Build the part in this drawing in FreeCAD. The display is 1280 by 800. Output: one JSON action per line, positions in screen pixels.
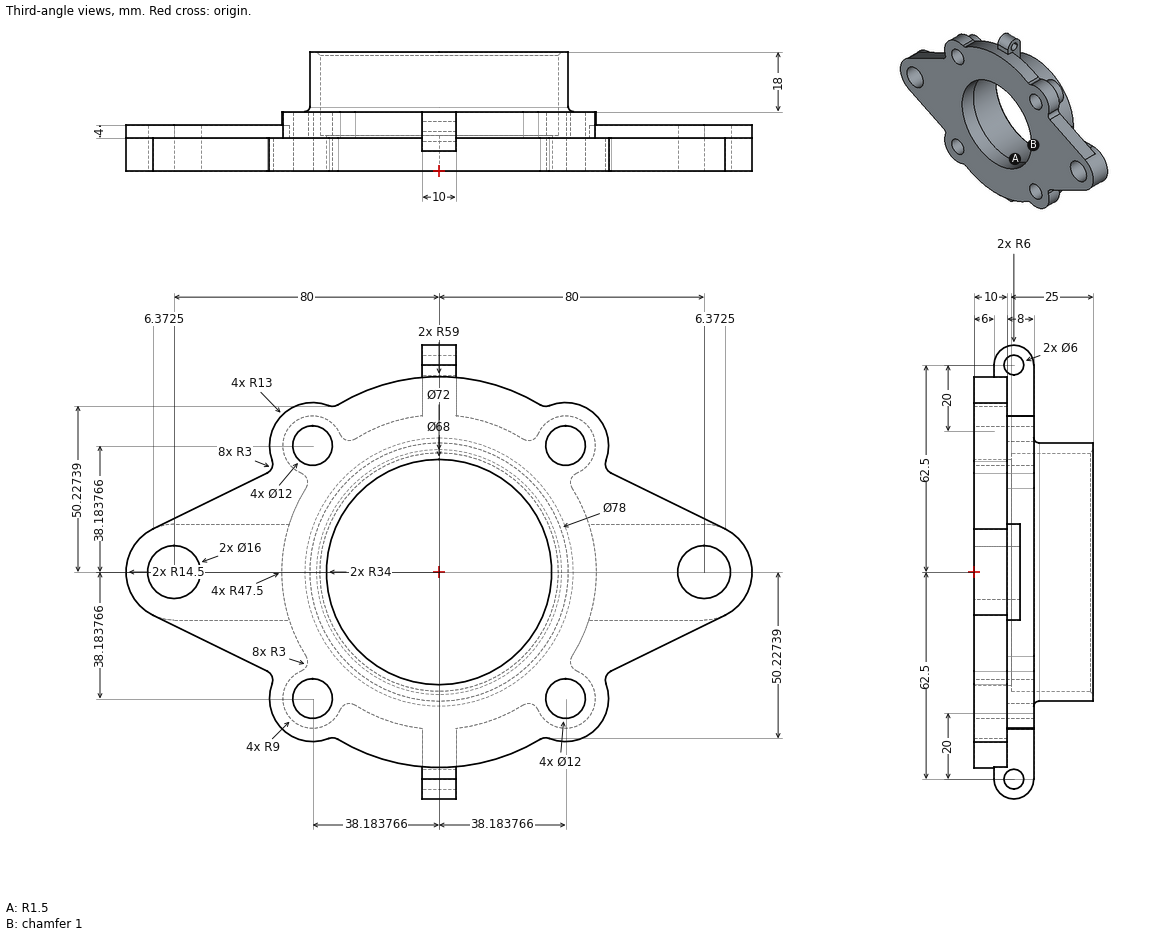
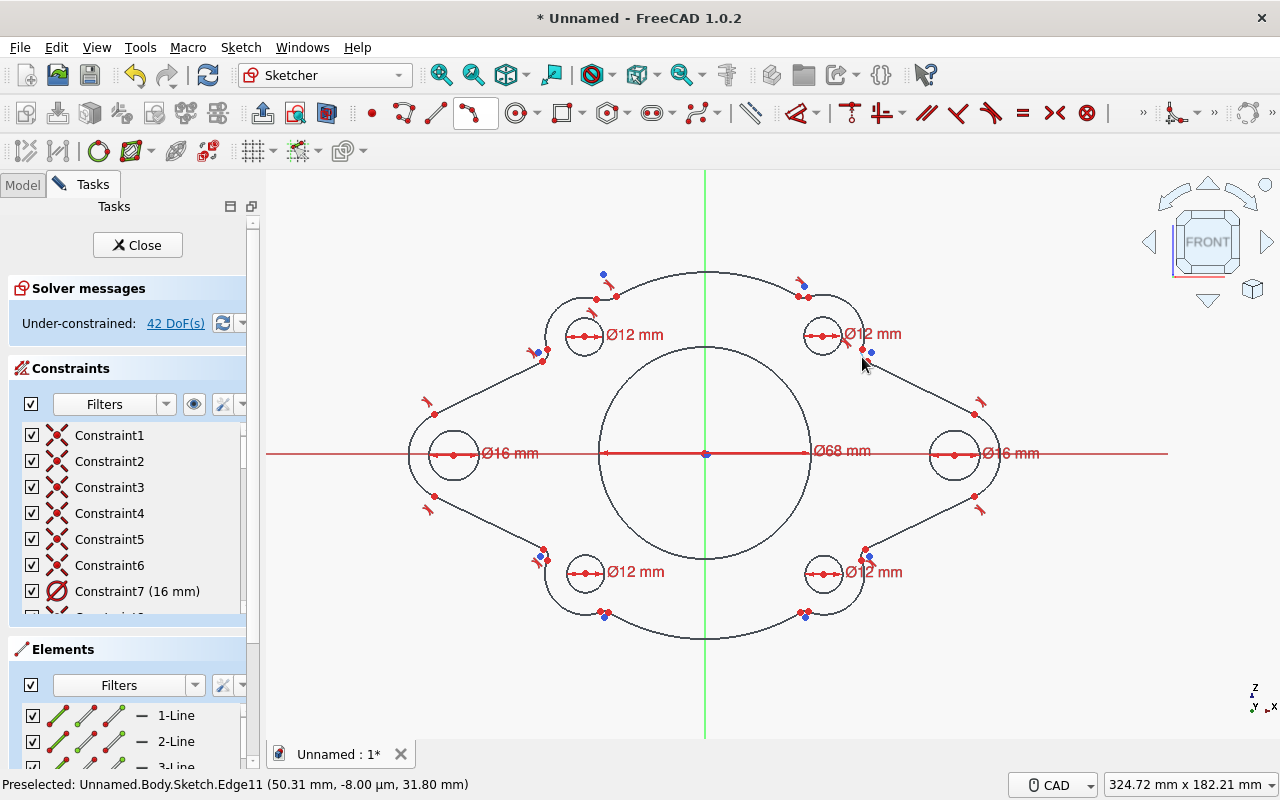
{"action": "scroll", "coordinate": [862, 554], "scroll_direction": "up", "scroll_amount": 4}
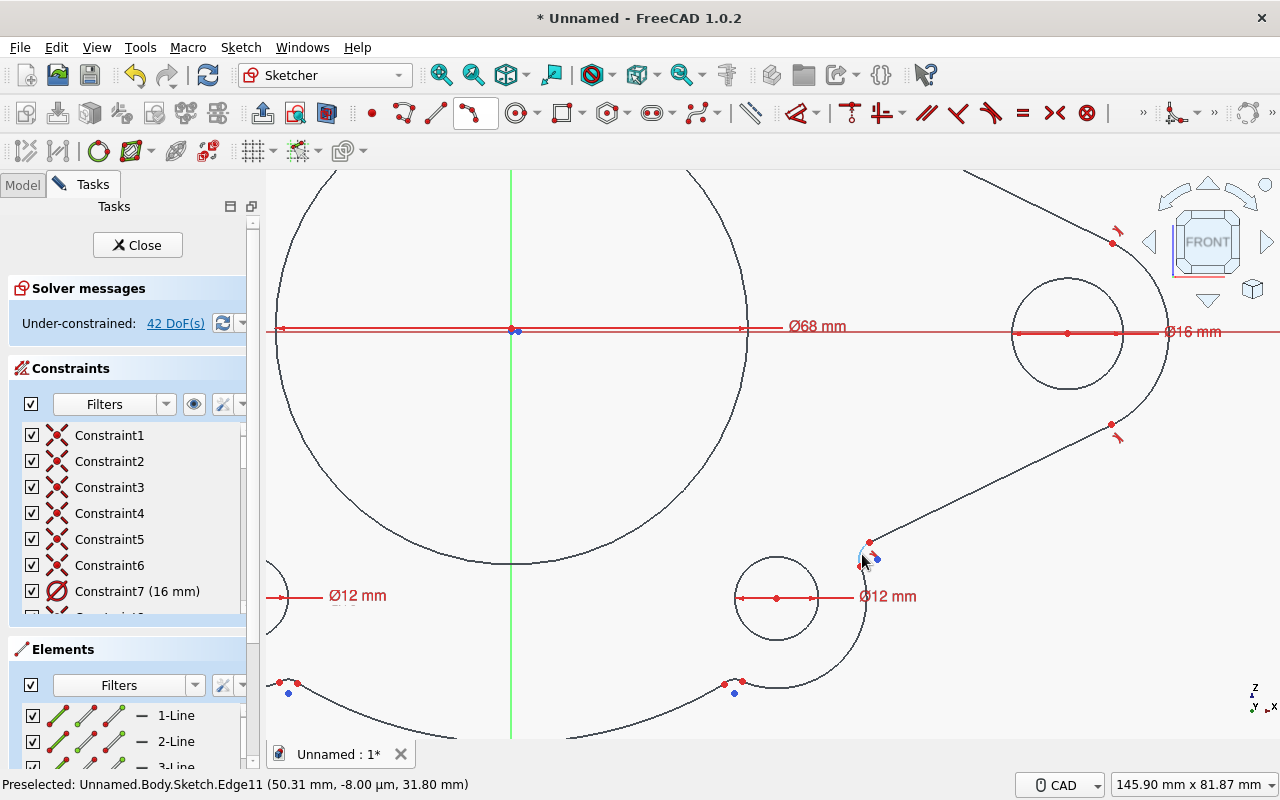
{"action": "left_click", "coordinate": [860, 553]}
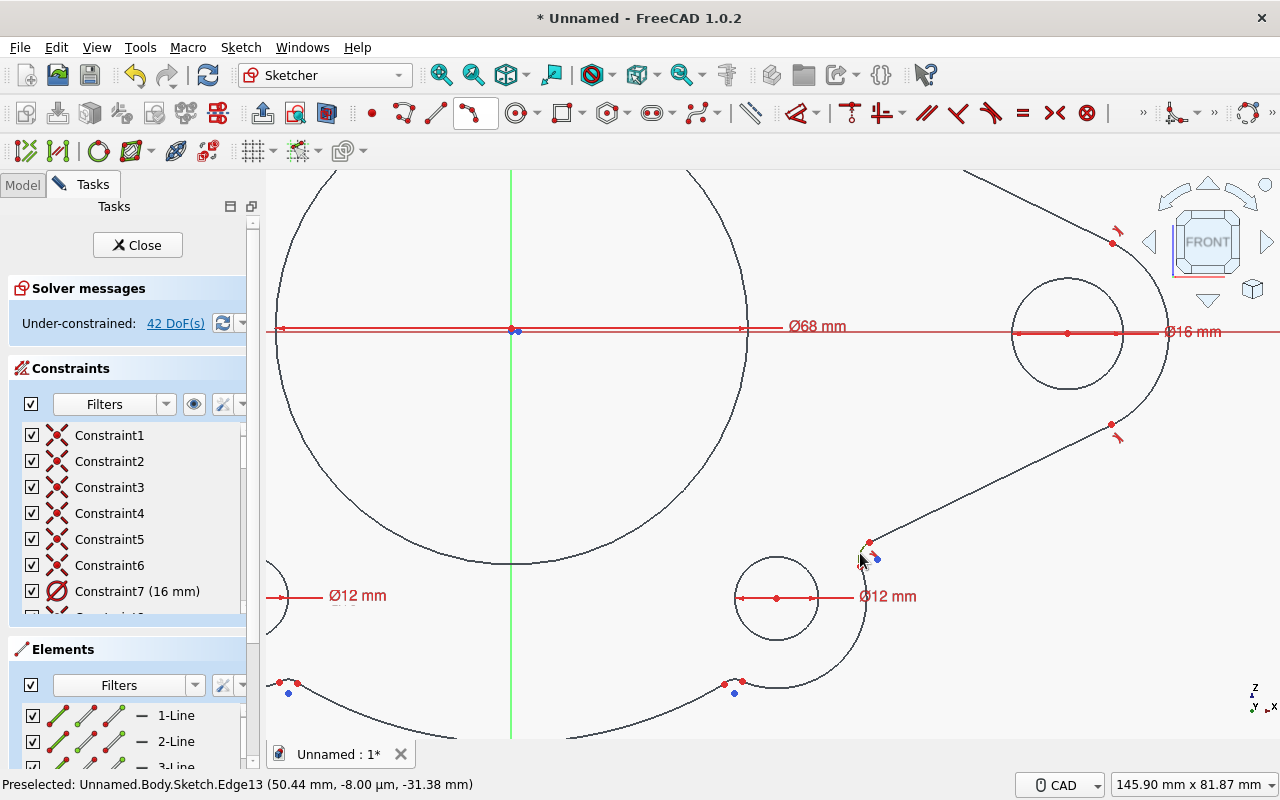
{"action": "left_click", "coordinate": [804, 684]}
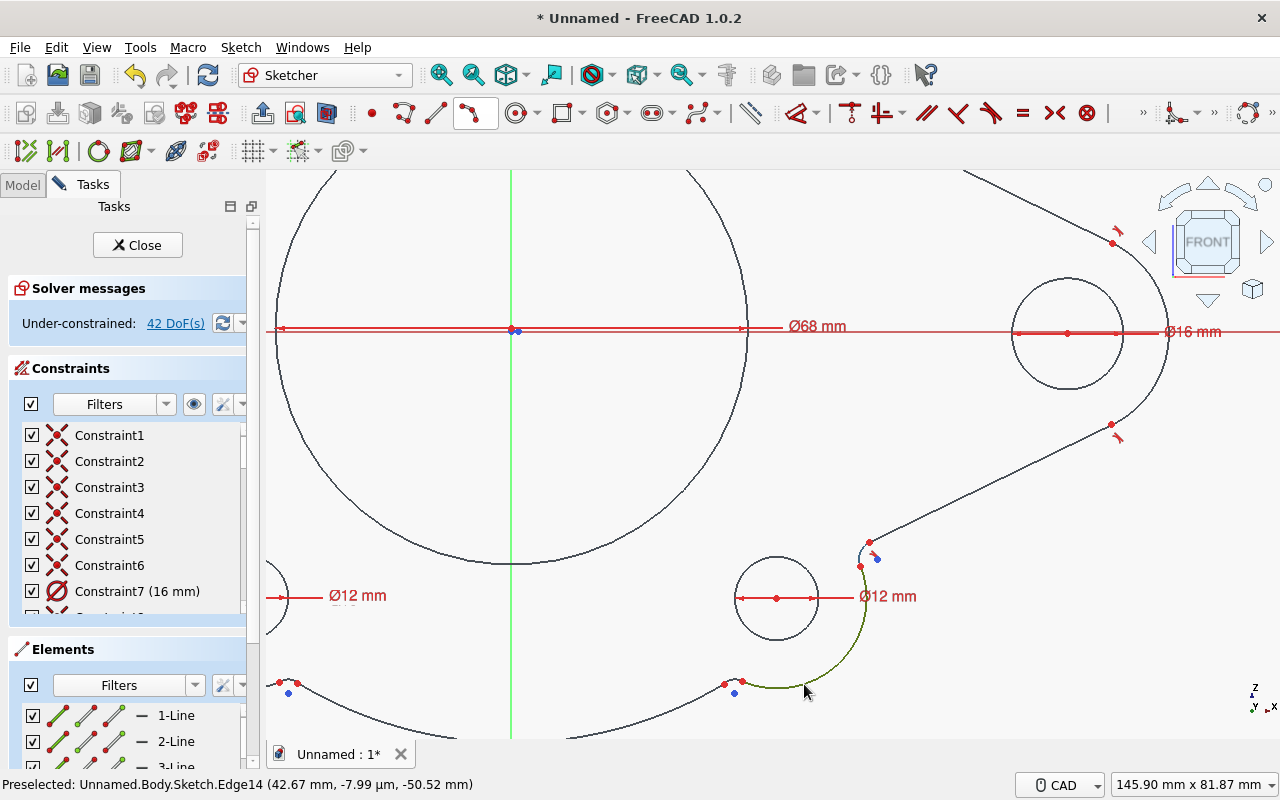
{"action": "left_click", "coordinate": [992, 114]}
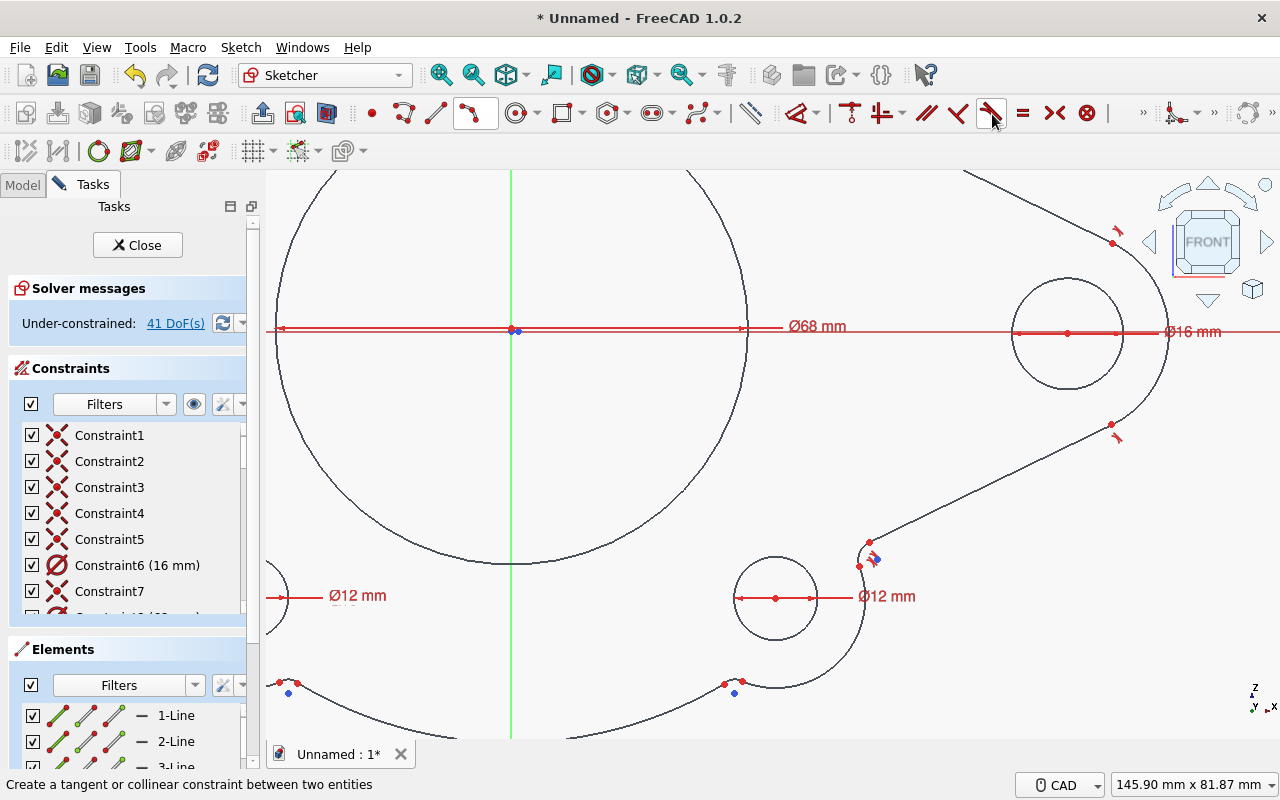
{"action": "left_click", "coordinate": [803, 684]}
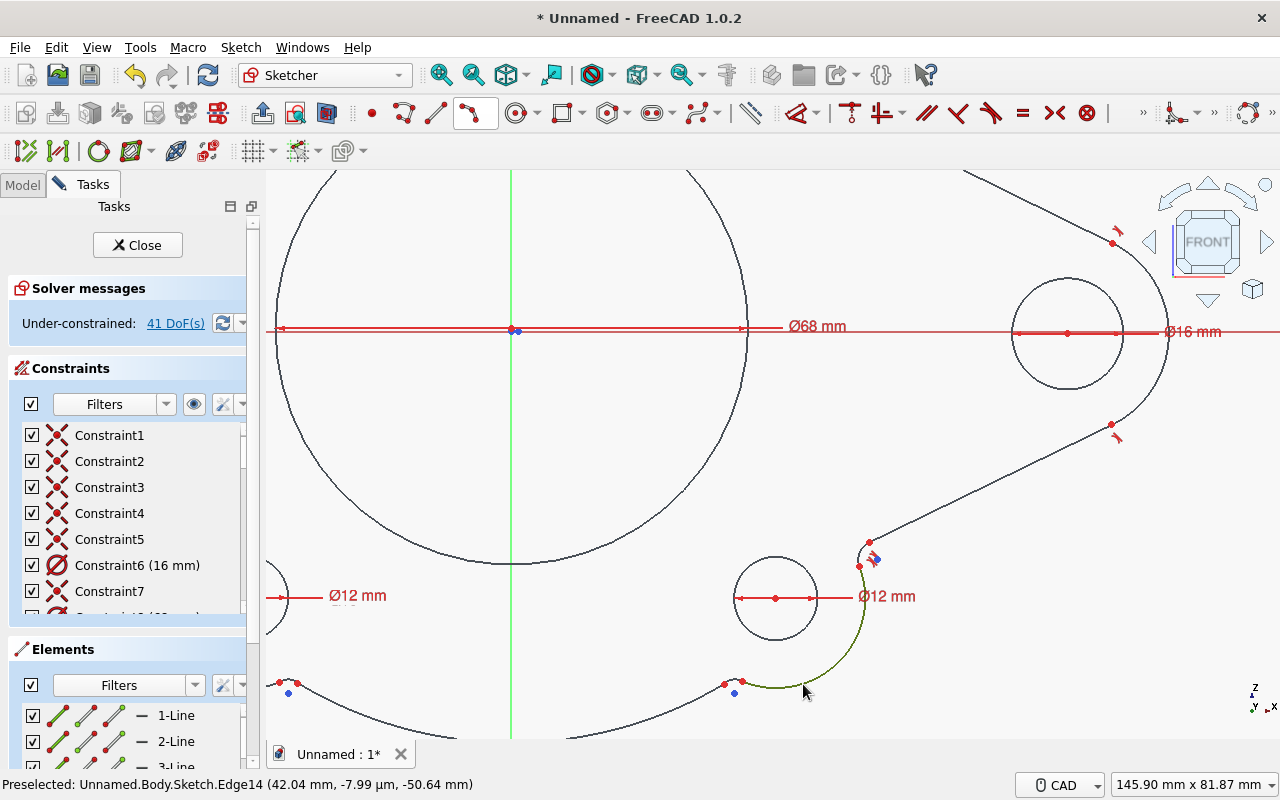
{"action": "scroll", "coordinate": [733, 680], "scroll_direction": "up", "scroll_amount": 2}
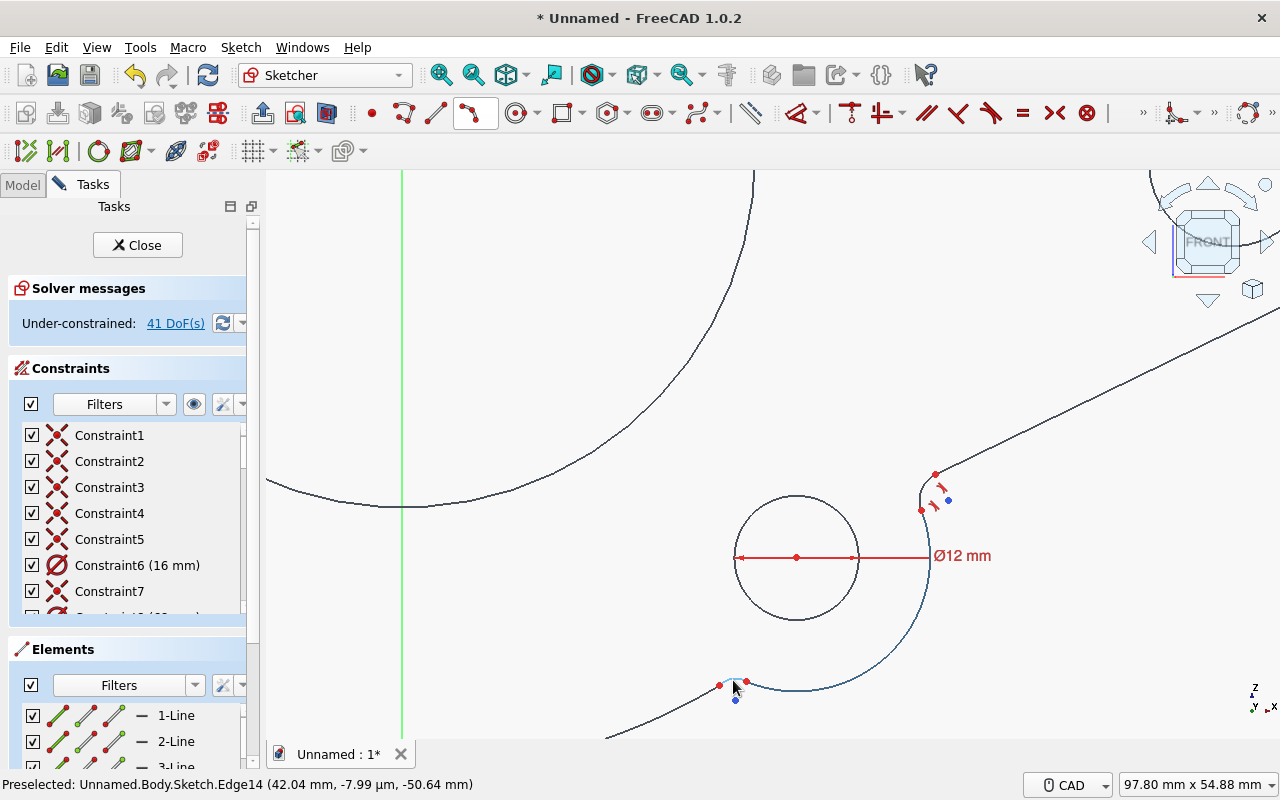
{"action": "left_click", "coordinate": [733, 679]}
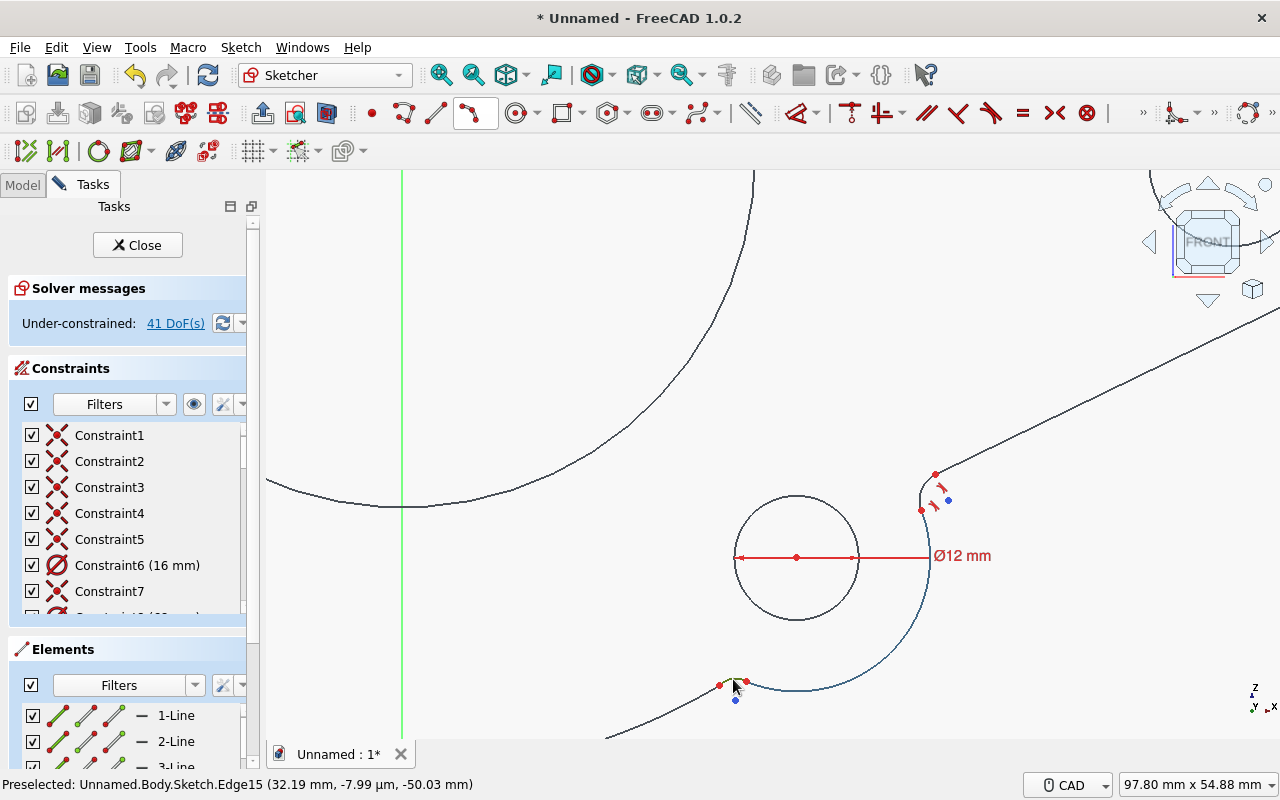
{"action": "left_click", "coordinate": [992, 114]}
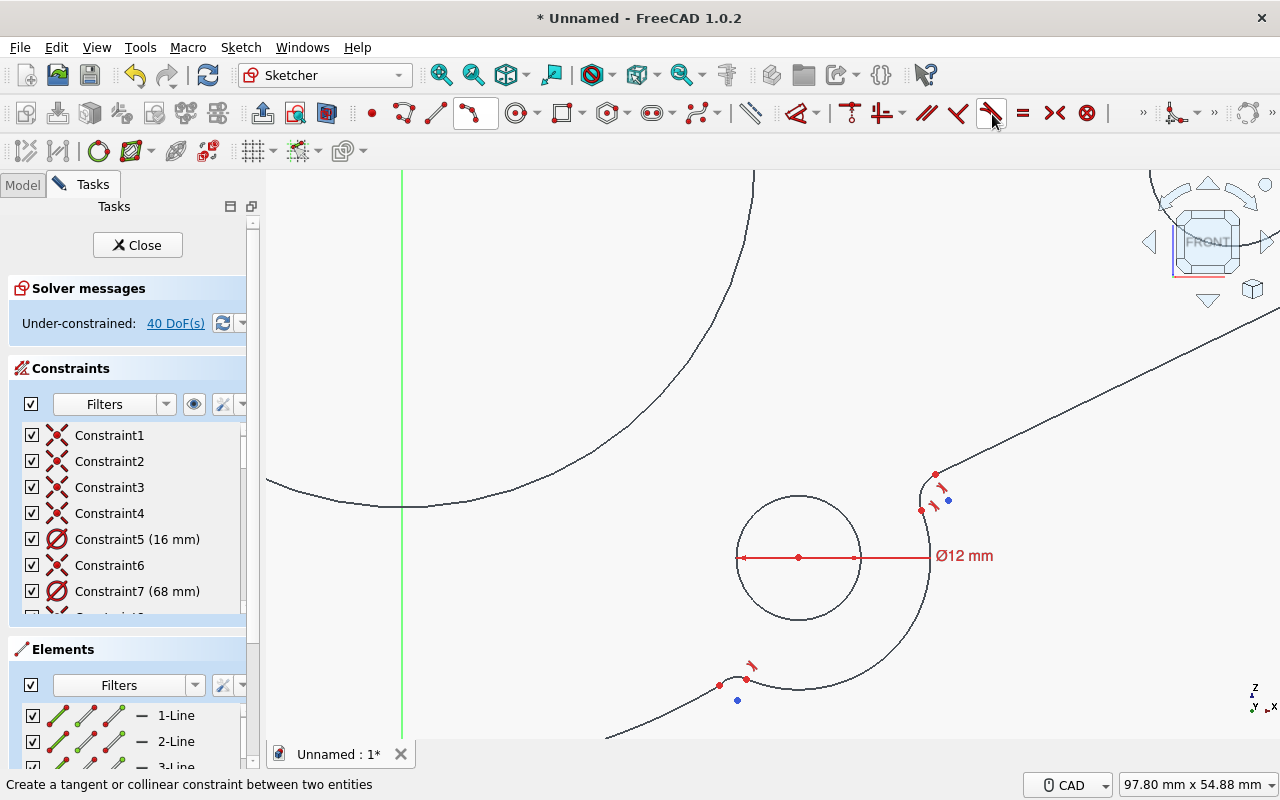
{"action": "left_click", "coordinate": [732, 678]}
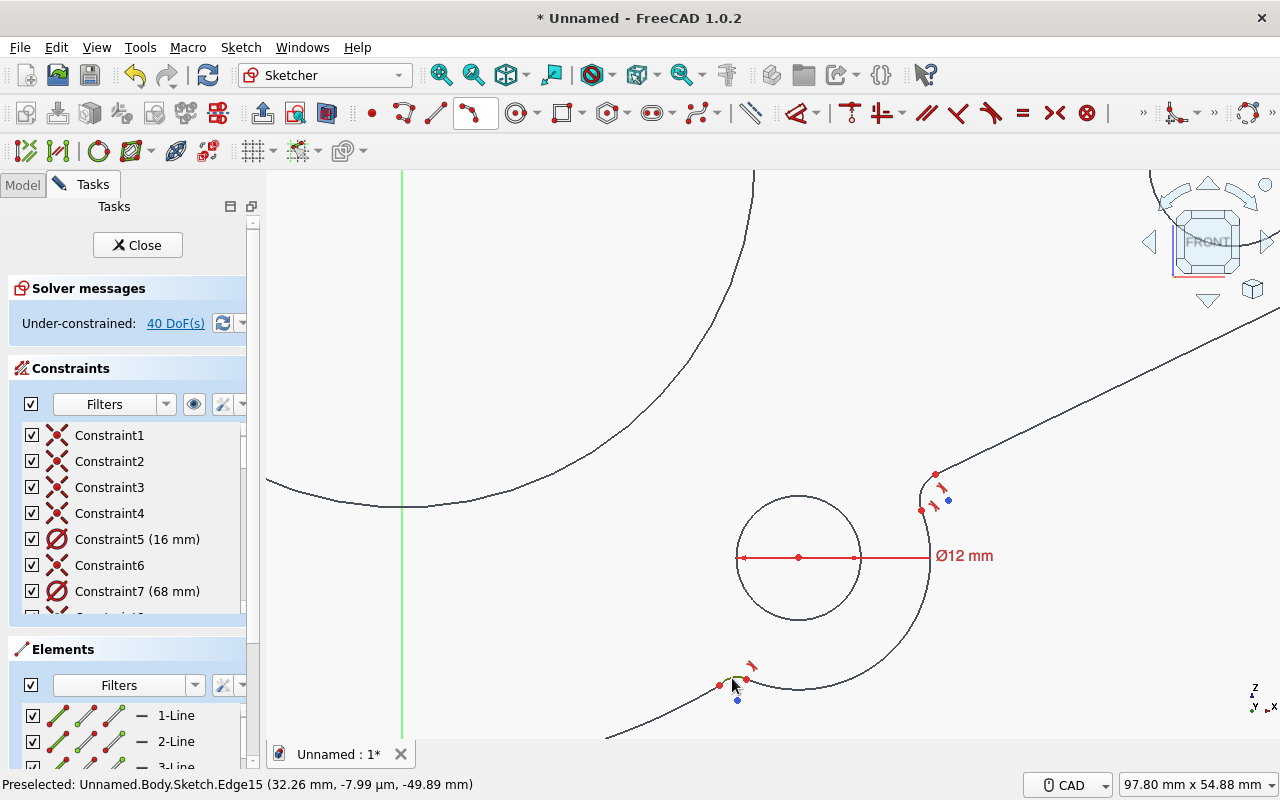
{"action": "scroll", "coordinate": [835, 581], "scroll_direction": "down", "scroll_amount": 6}